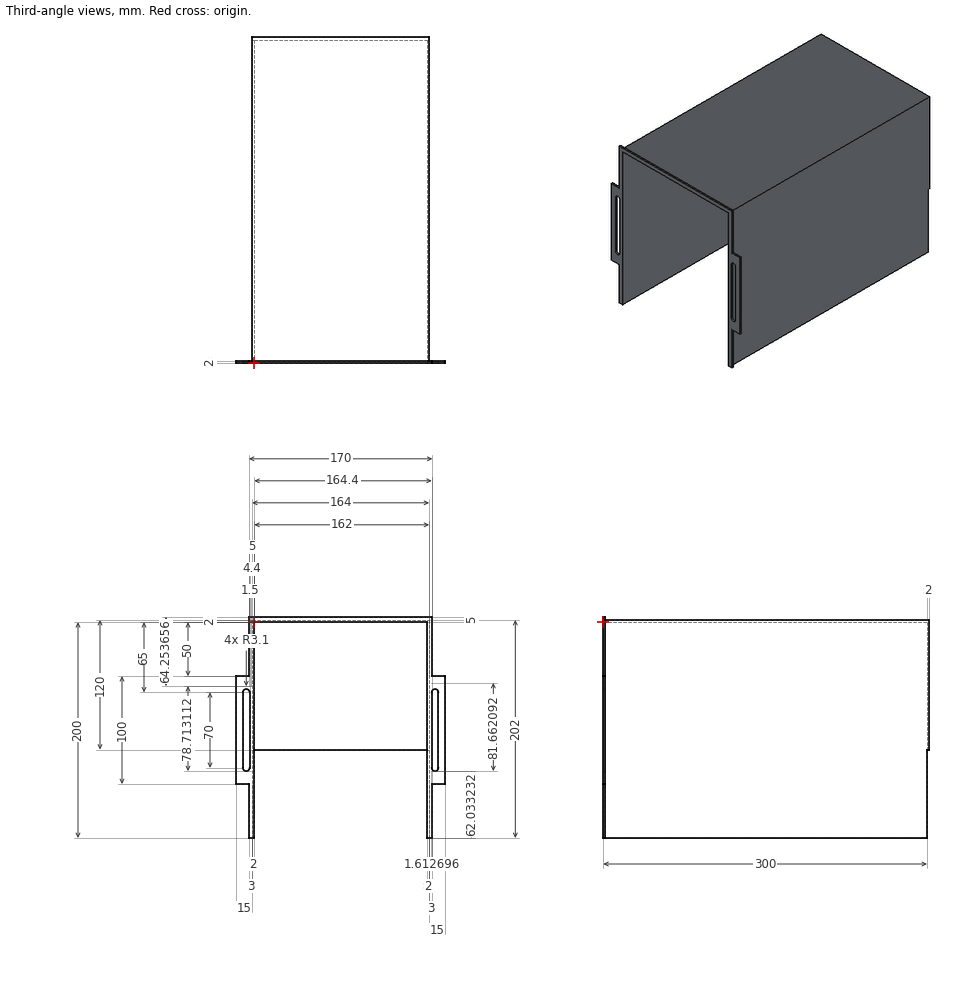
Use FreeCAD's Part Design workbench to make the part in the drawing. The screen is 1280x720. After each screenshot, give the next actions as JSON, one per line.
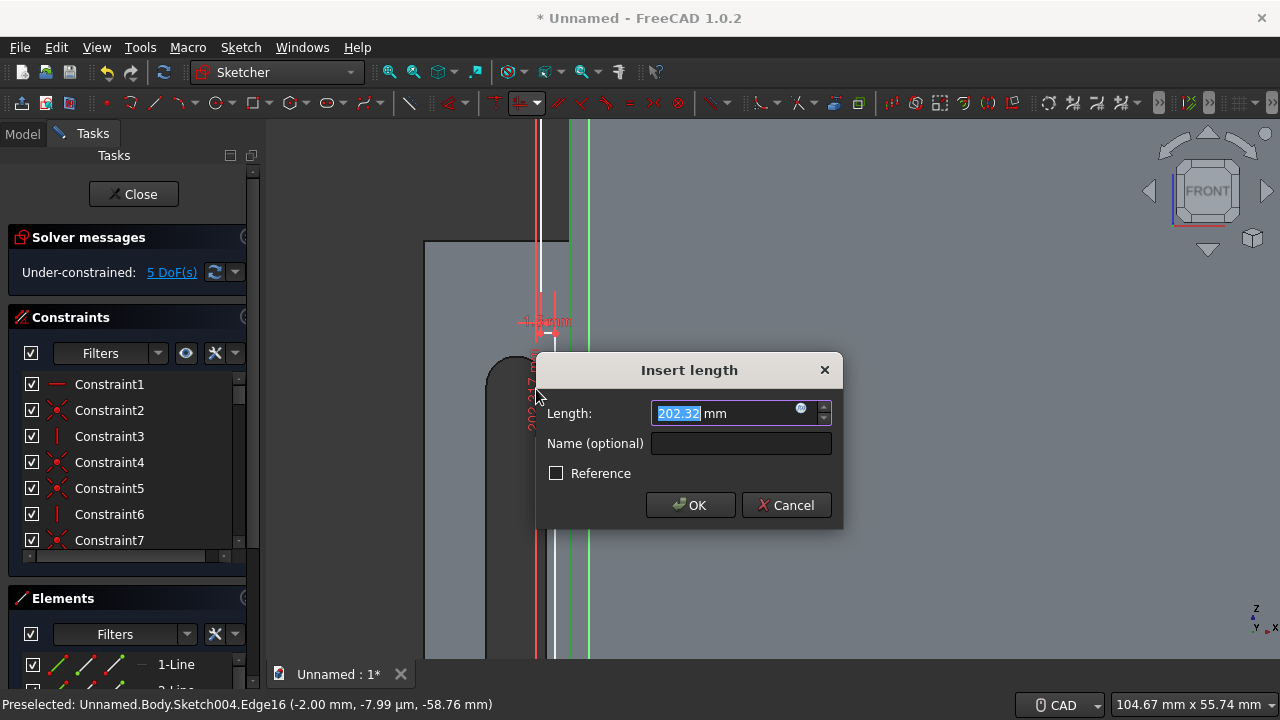
{"action": "type", "text": "202"}
{"action": "key", "text": "Return"}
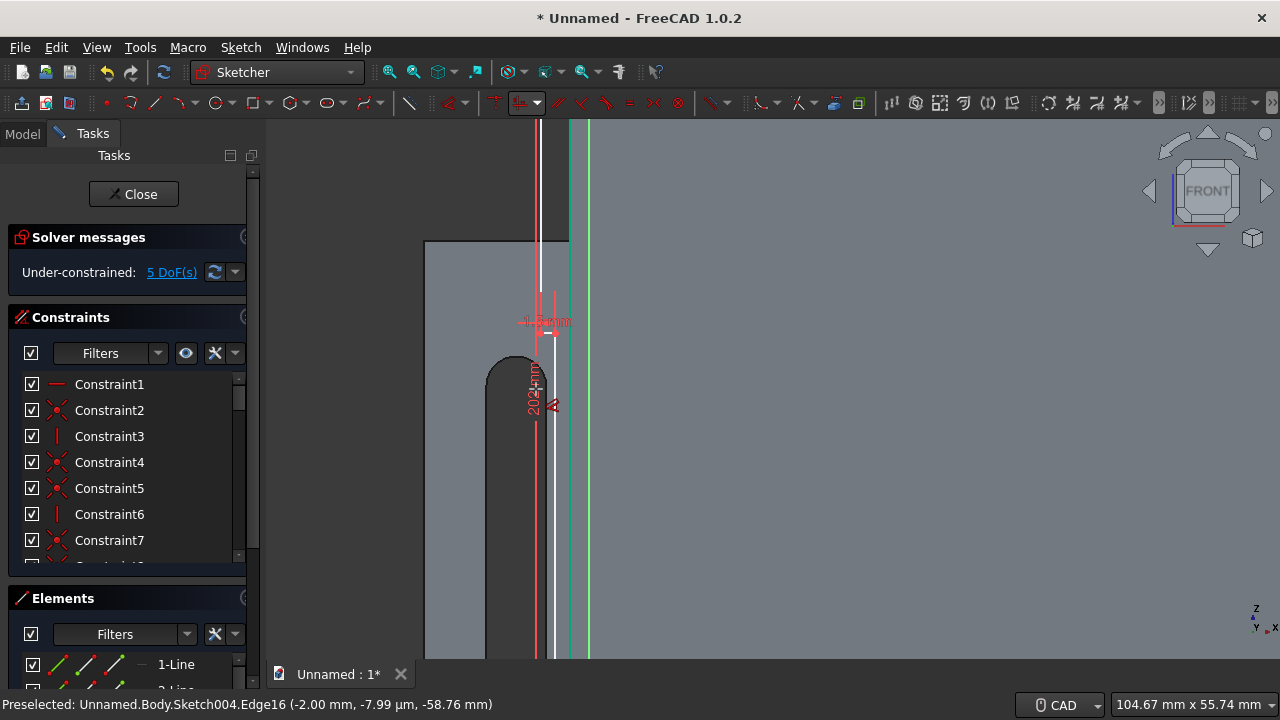
{"action": "scroll", "coordinate": [574, 327], "scroll_direction": "down", "scroll_amount": 9}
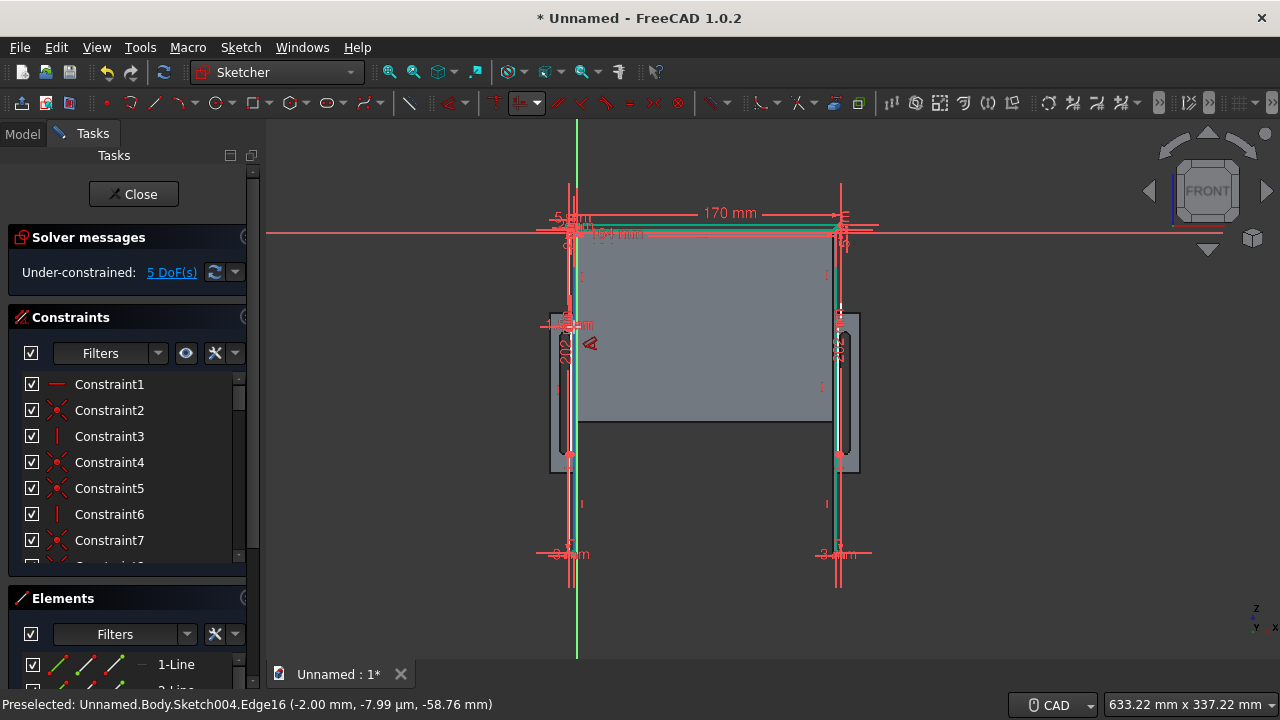
{"action": "scroll", "coordinate": [840, 454], "scroll_direction": "up", "scroll_amount": 14}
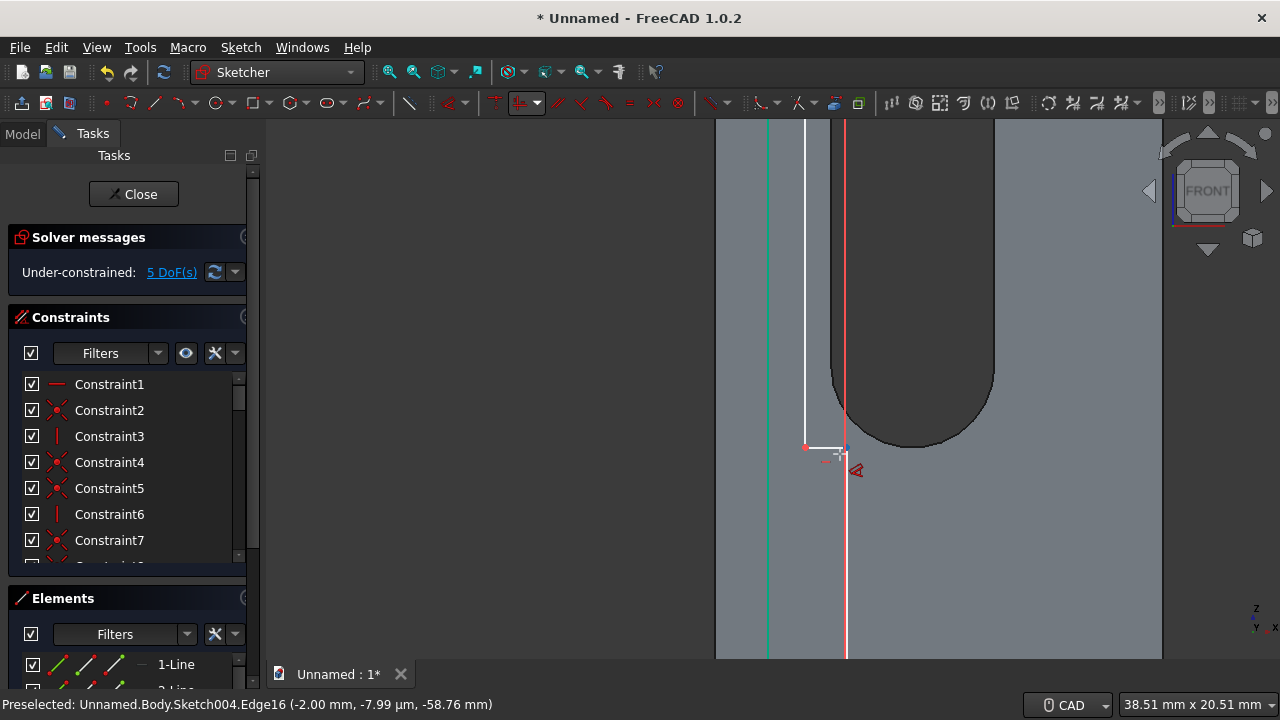
{"action": "left_click", "coordinate": [826, 448]}
{"action": "left_click", "coordinate": [826, 482]}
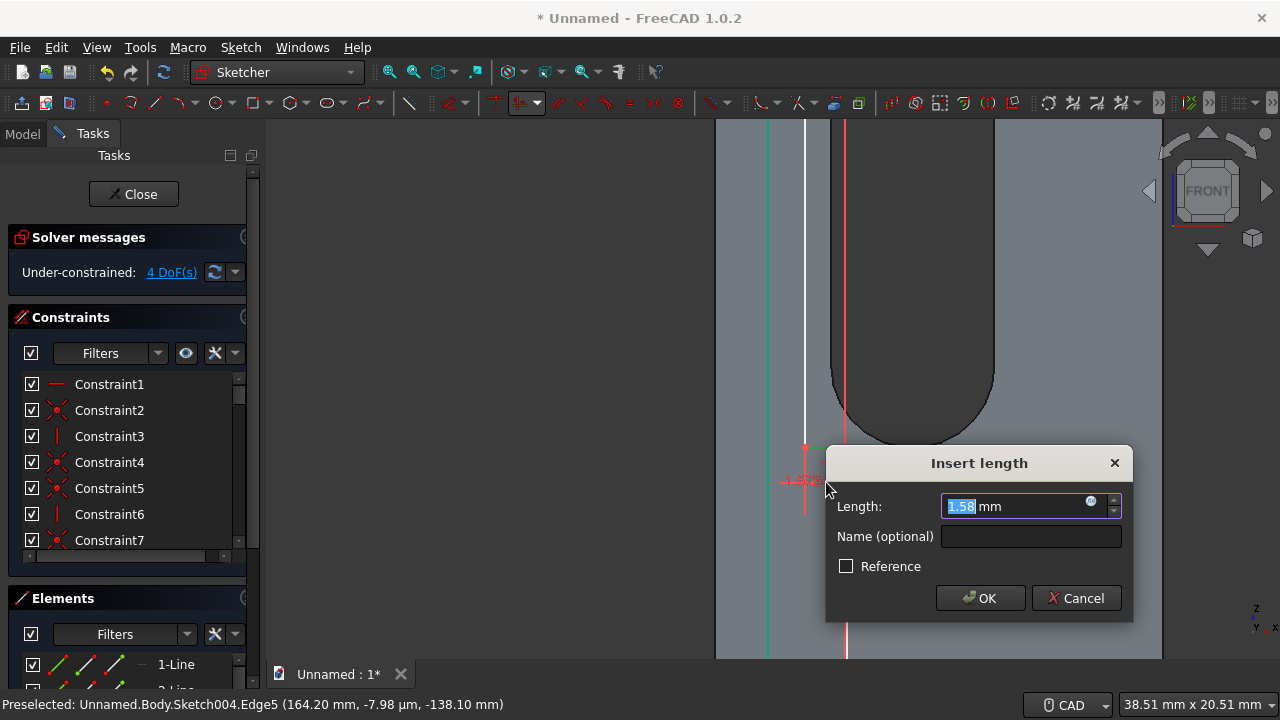
{"action": "type", "text": "1.612696"}
{"action": "key", "text": "Return"}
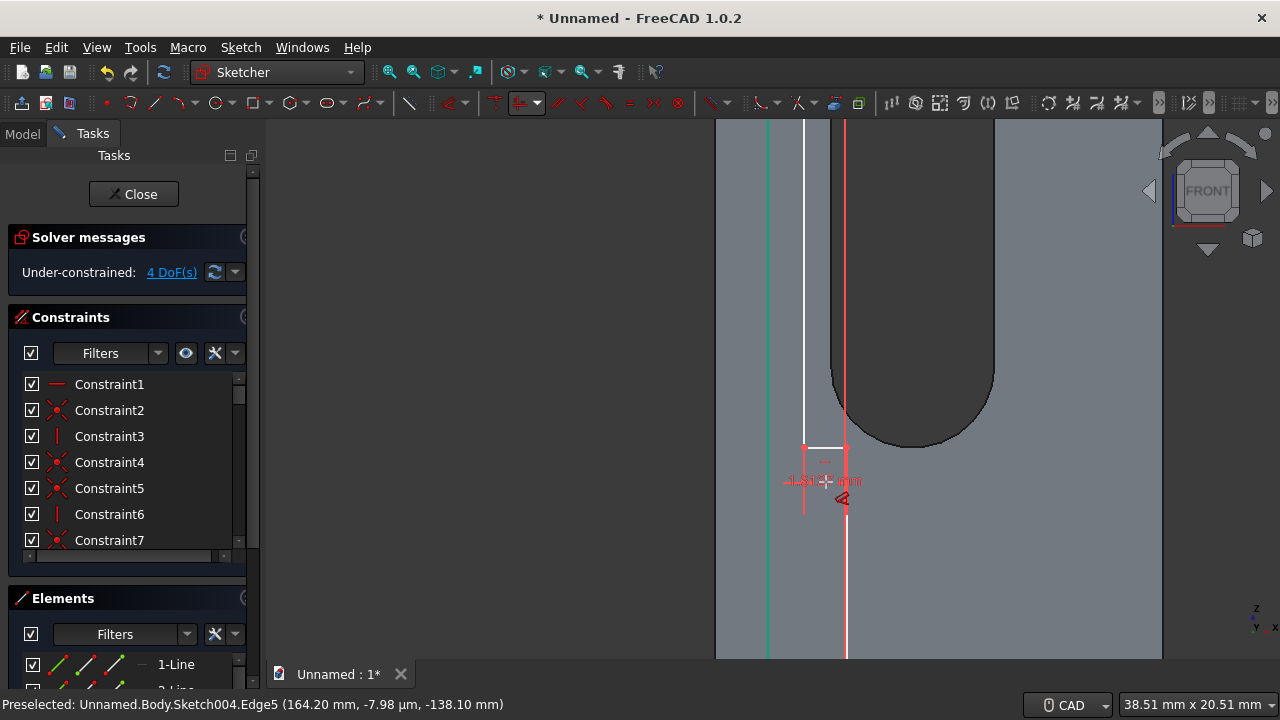
{"action": "scroll", "coordinate": [840, 454], "scroll_direction": "down", "scroll_amount": 14}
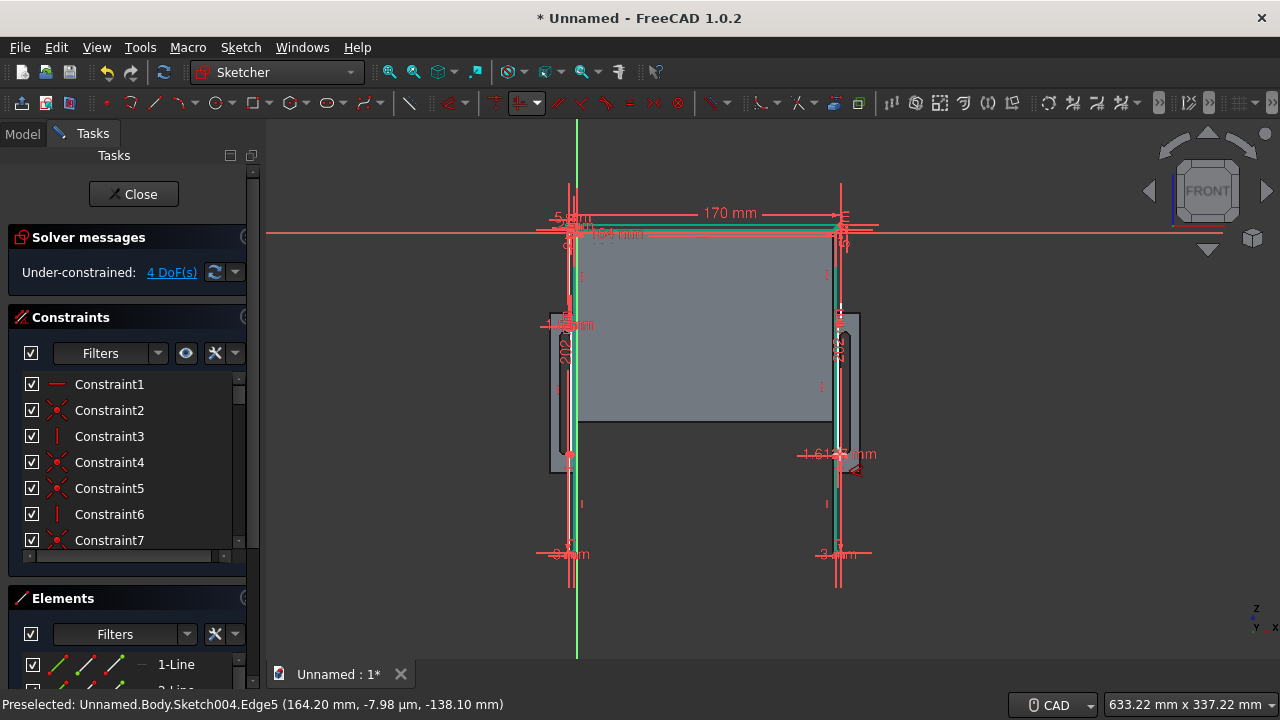
{"action": "scroll", "coordinate": [841, 524], "scroll_direction": "up", "scroll_amount": 6}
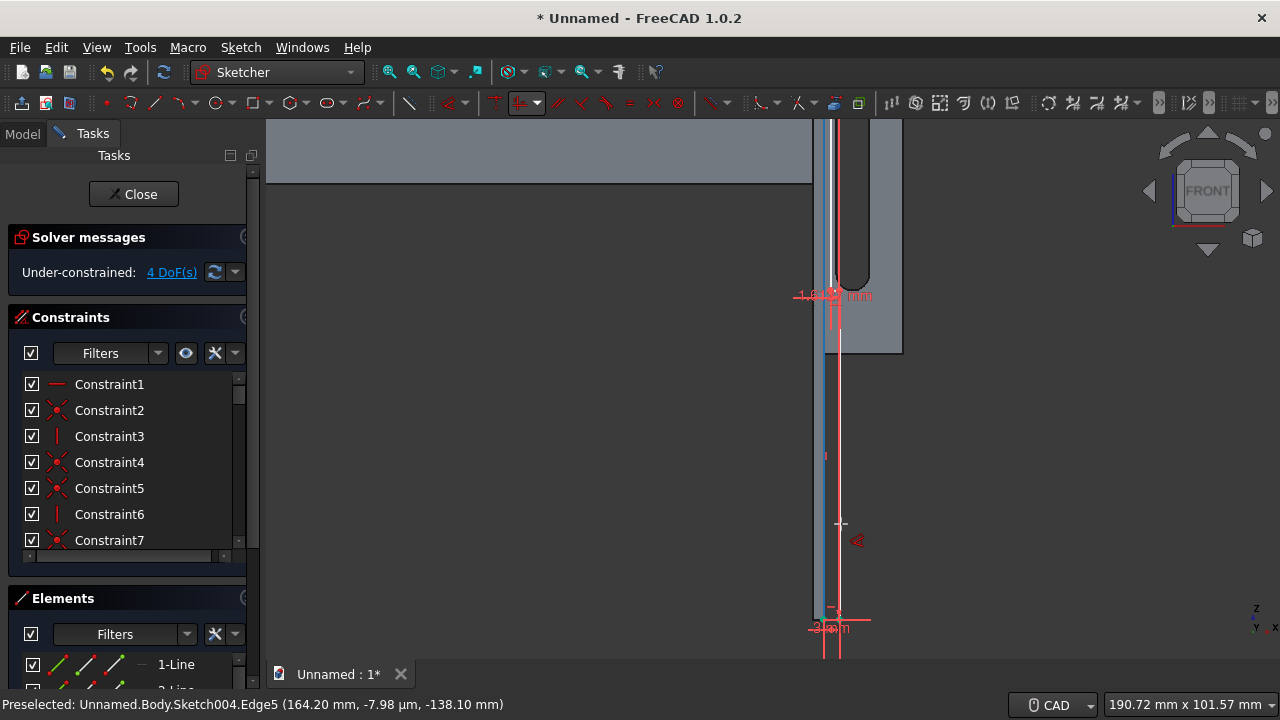
{"action": "left_click", "coordinate": [840, 521]}
{"action": "left_click", "coordinate": [874, 455]}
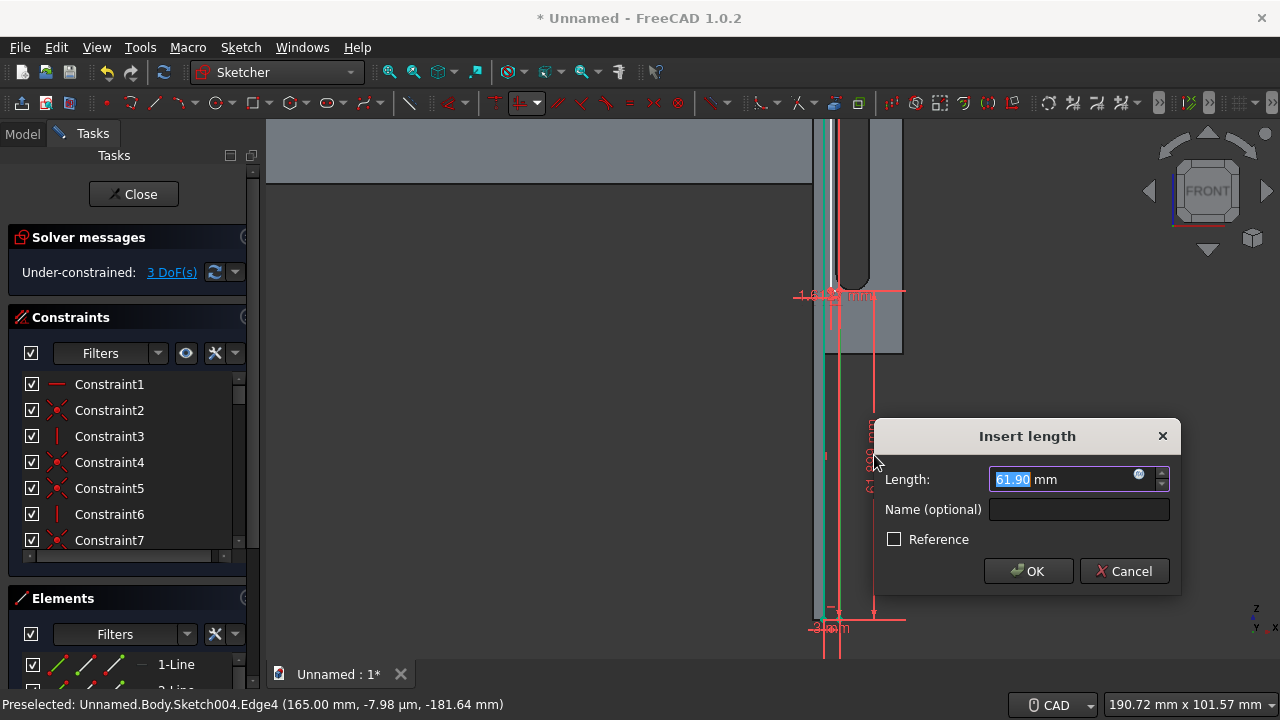
{"action": "type", "text": "62.033232"}
{"action": "key", "text": "Return"}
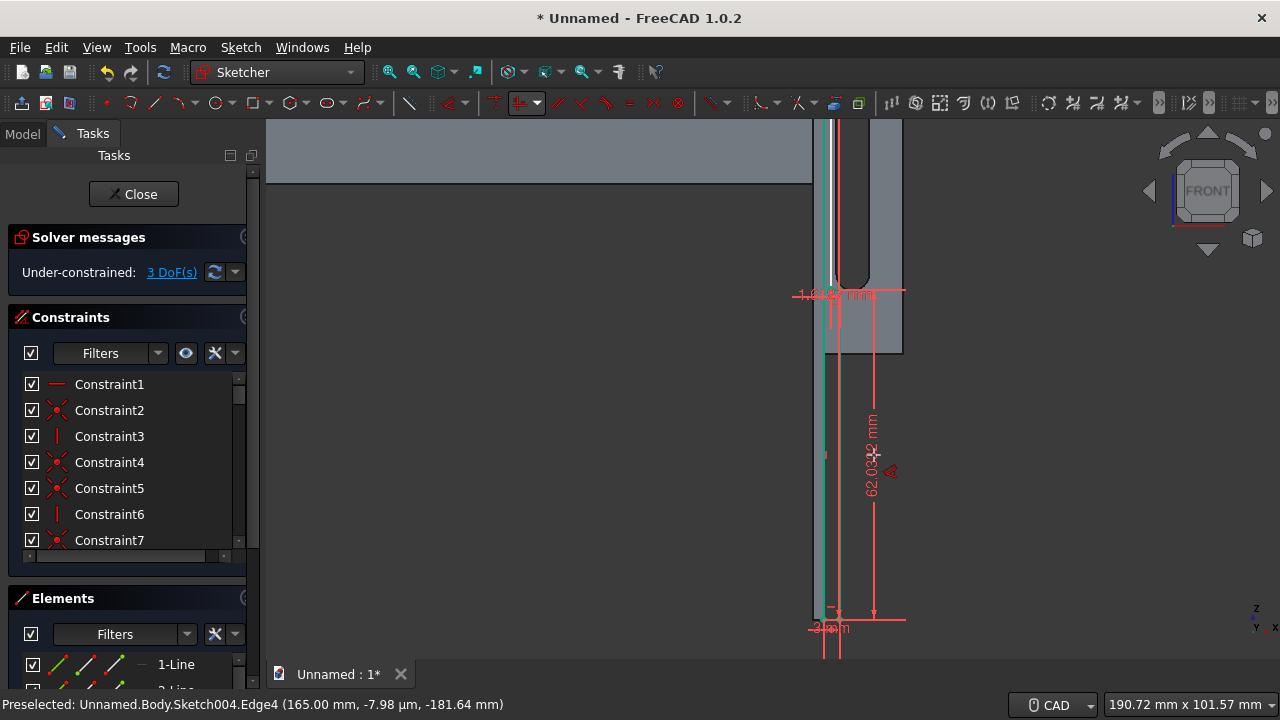
{"action": "scroll", "coordinate": [831, 160], "scroll_direction": "up", "scroll_amount": 4}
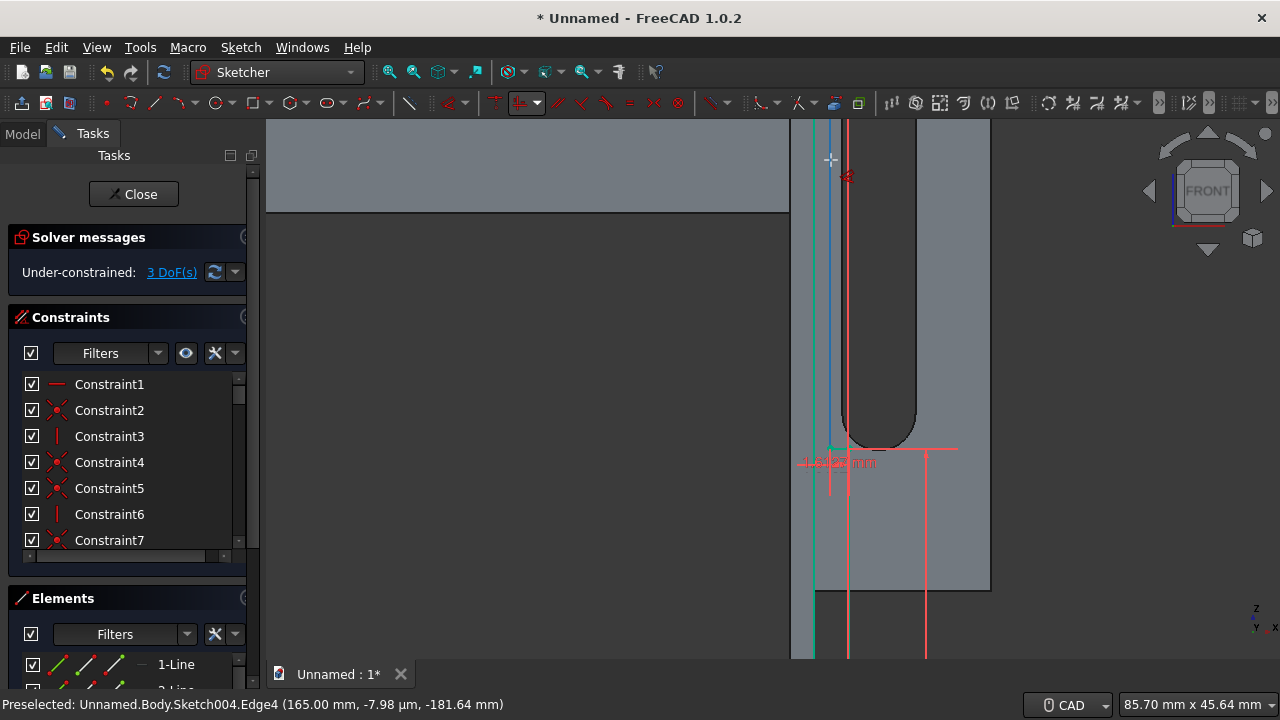
{"action": "left_click", "coordinate": [830, 159]}
{"action": "left_click", "coordinate": [864, 298]}